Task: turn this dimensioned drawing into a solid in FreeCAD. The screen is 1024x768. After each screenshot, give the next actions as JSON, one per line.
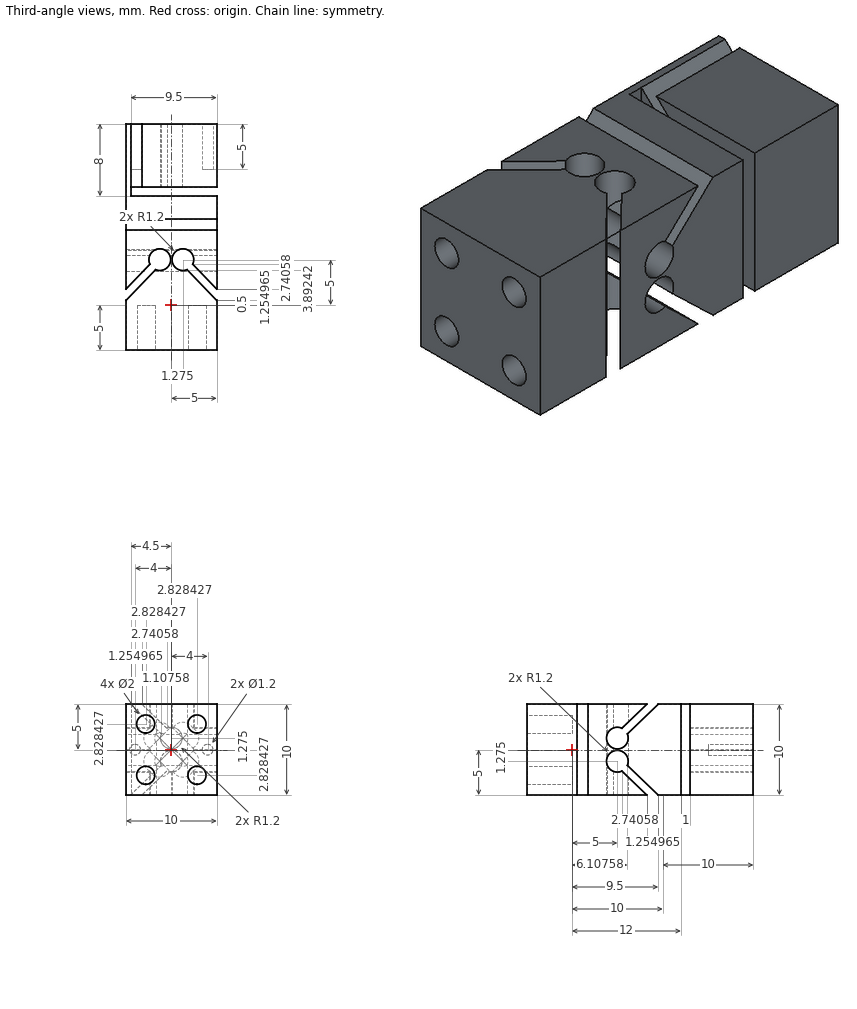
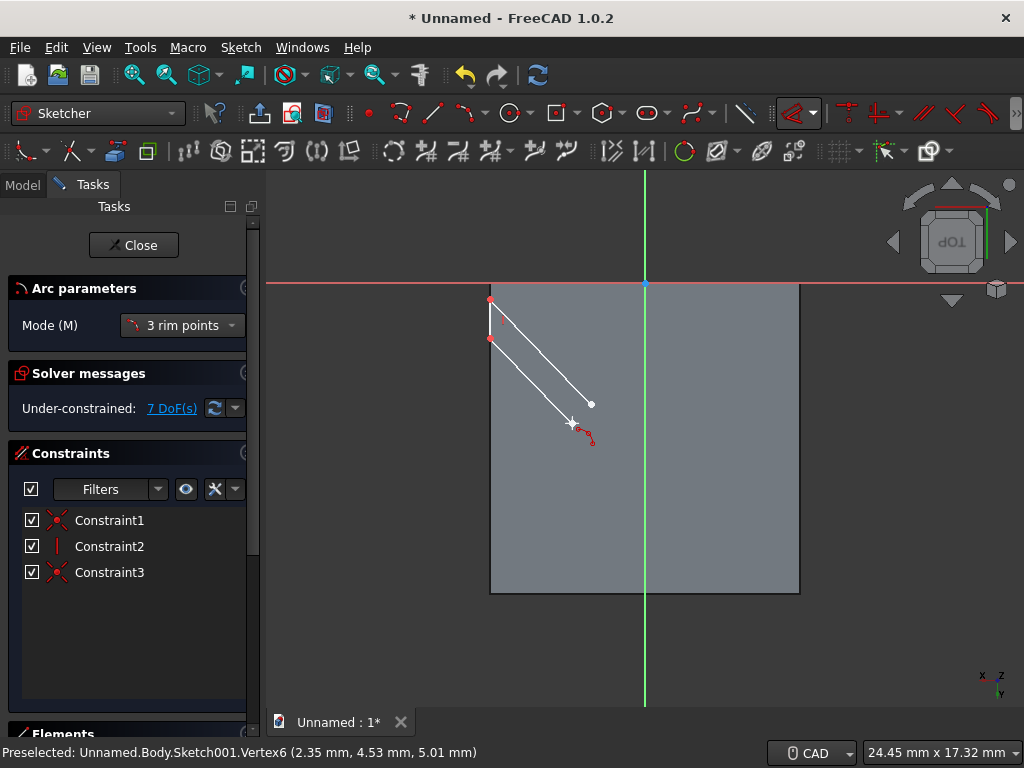
{"action": "left_click", "coordinate": [572, 424]}
{"action": "left_click", "coordinate": [591, 405]}
{"action": "left_click", "coordinate": [613, 475]}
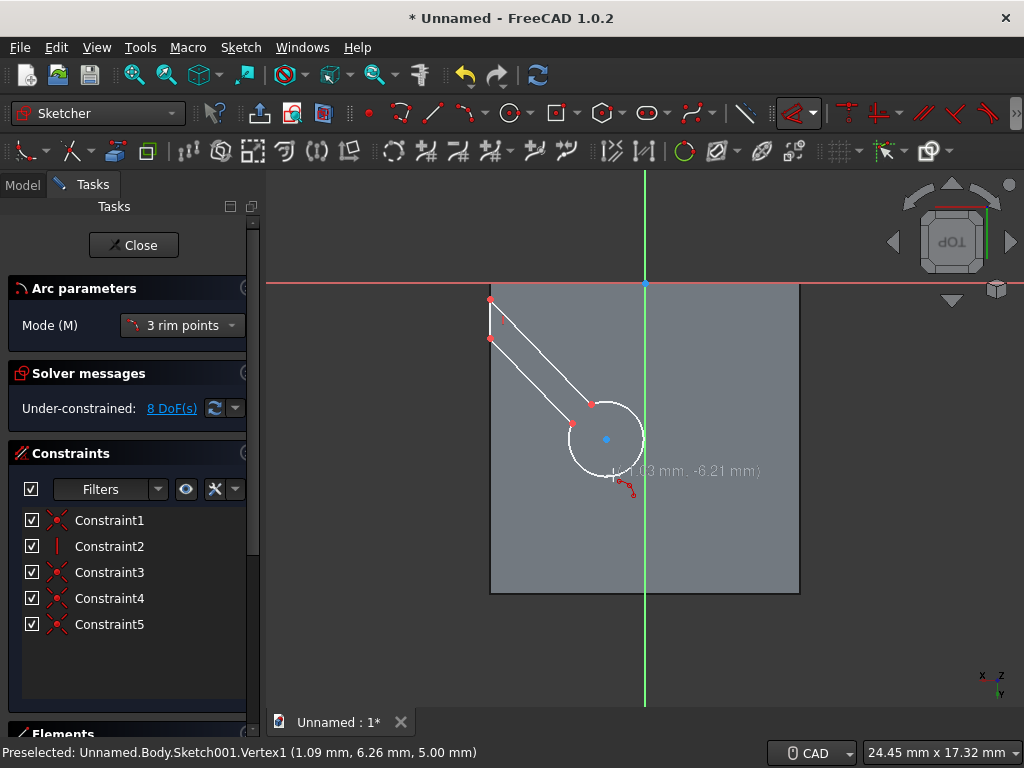
{"action": "left_click", "coordinate": [402, 114]}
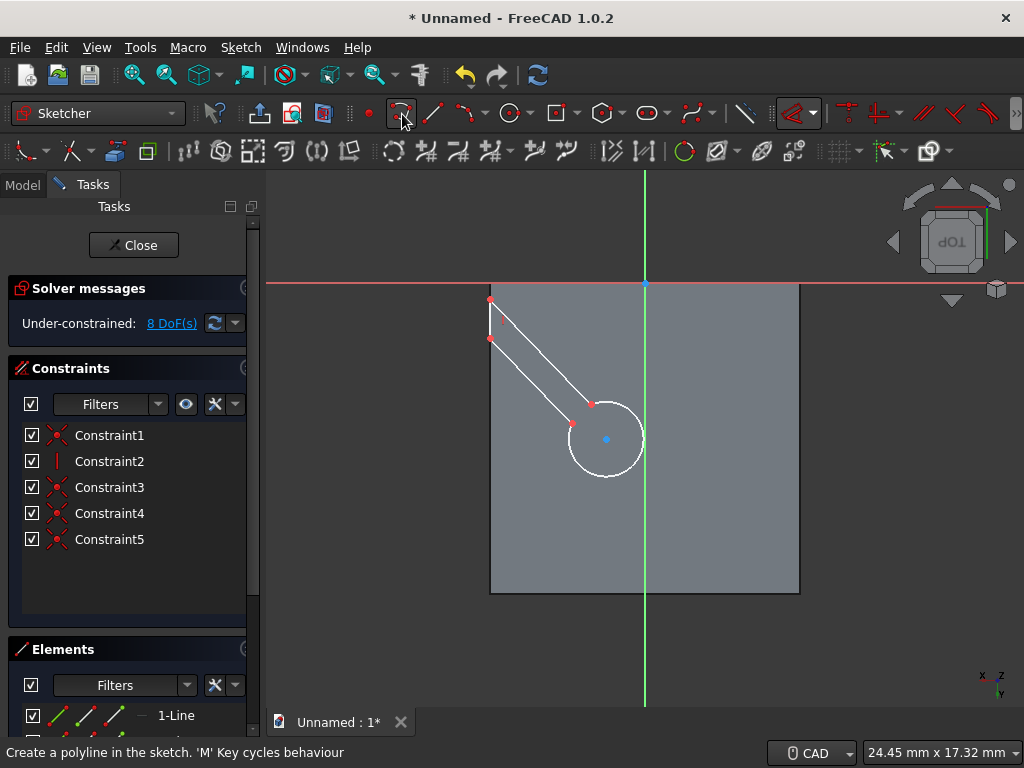
{"action": "left_click", "coordinate": [718, 423]}
{"action": "left_click", "coordinate": [800, 338]}
{"action": "left_click", "coordinate": [800, 299]}
{"action": "left_click", "coordinate": [699, 404]}
{"action": "right_click", "coordinate": [699, 404]}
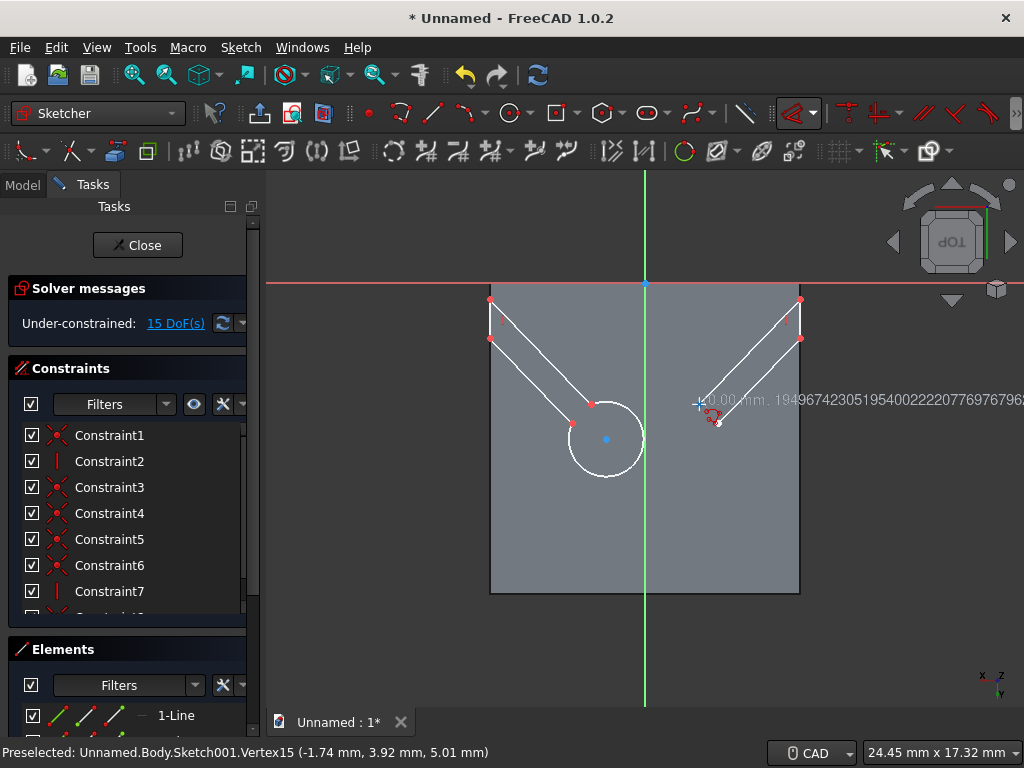
{"action": "key", "text": "g 3 a"}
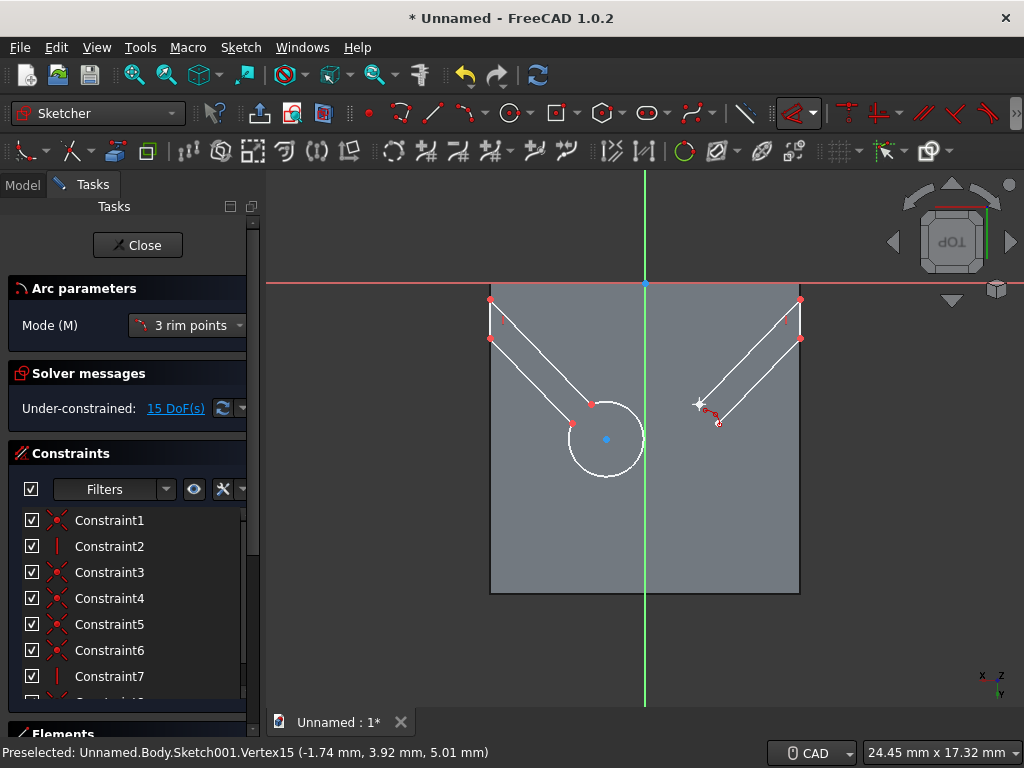
{"action": "left_click", "coordinate": [699, 405]}
{"action": "left_click", "coordinate": [718, 424]}
{"action": "left_click", "coordinate": [677, 475]}
{"action": "key", "text": "Escape"}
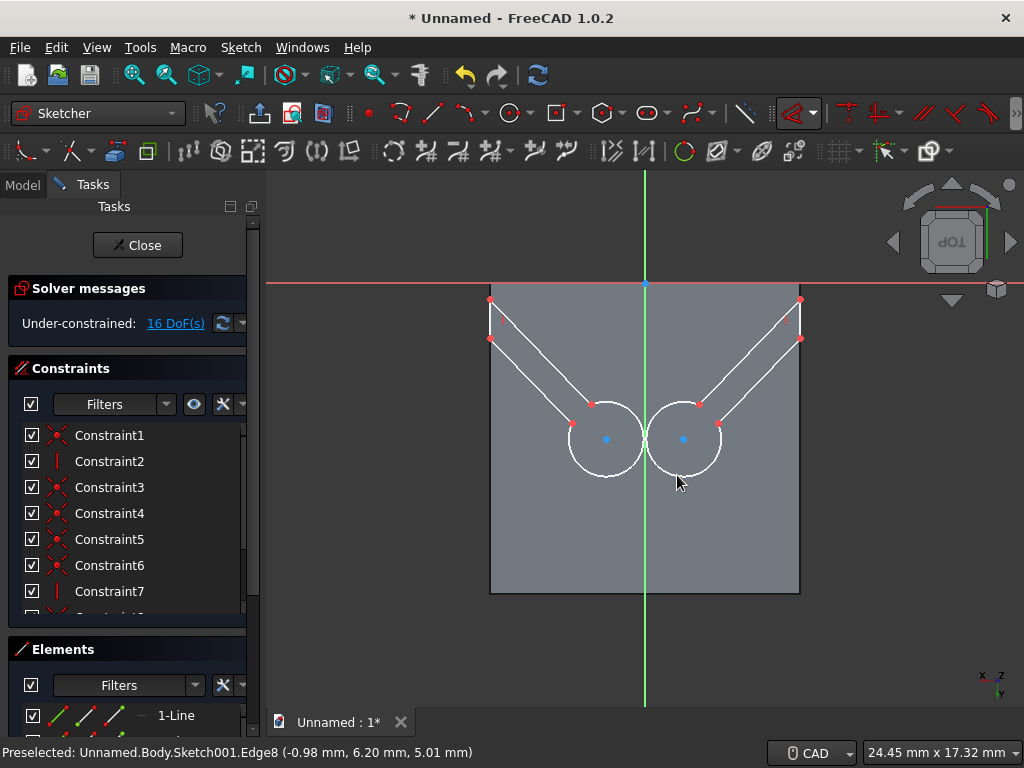
{"action": "left_click", "coordinate": [594, 475]}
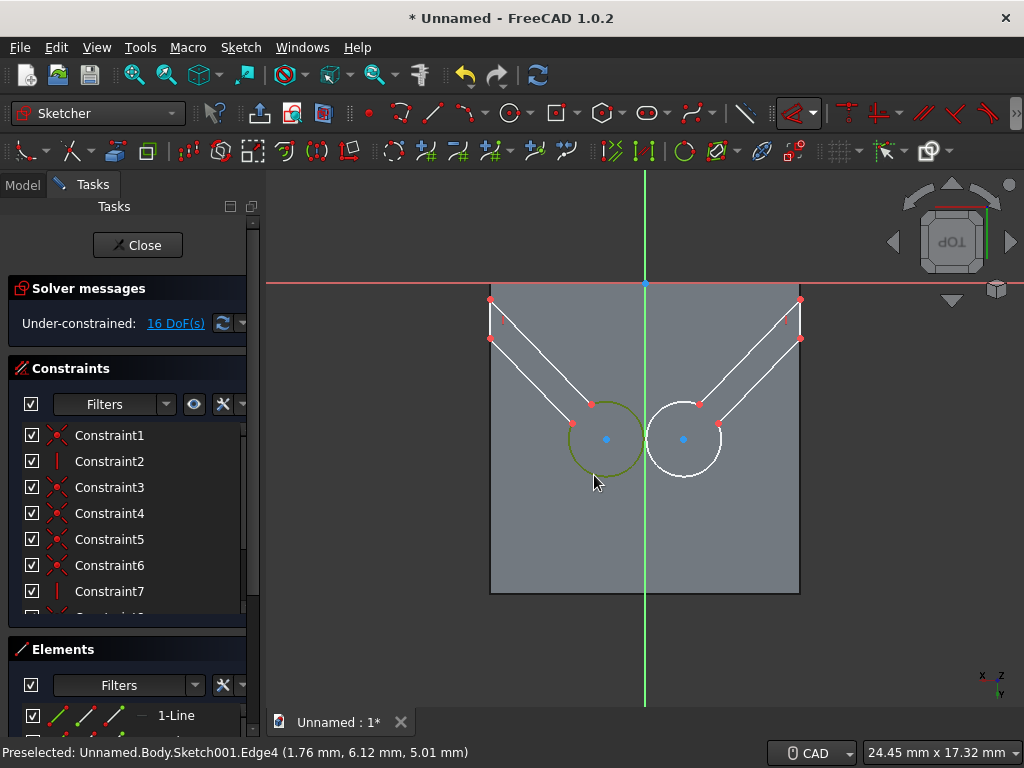
{"action": "left_click", "coordinate": [696, 475]}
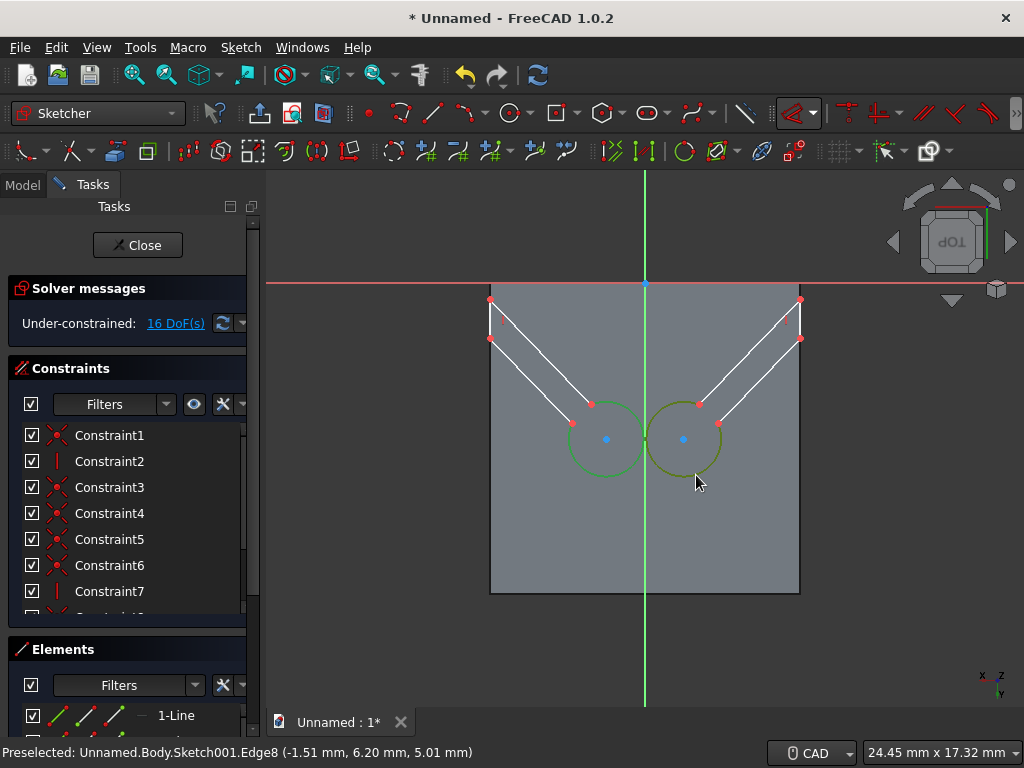
{"action": "key", "text": "e"}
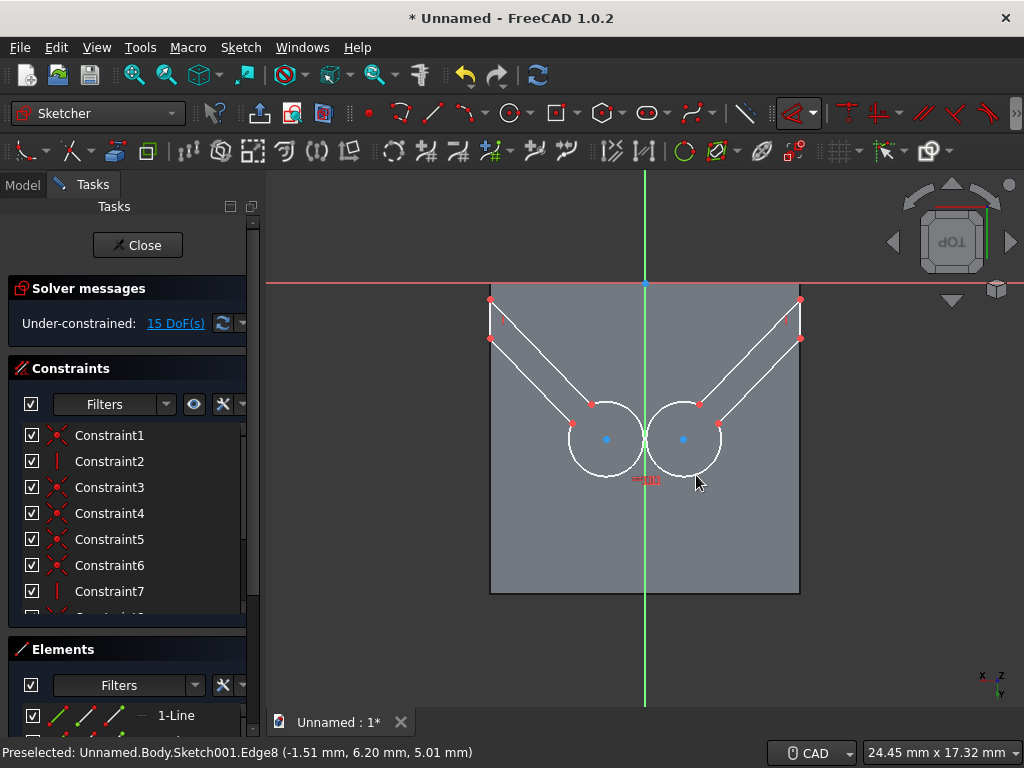
{"action": "left_click", "coordinate": [606, 439]}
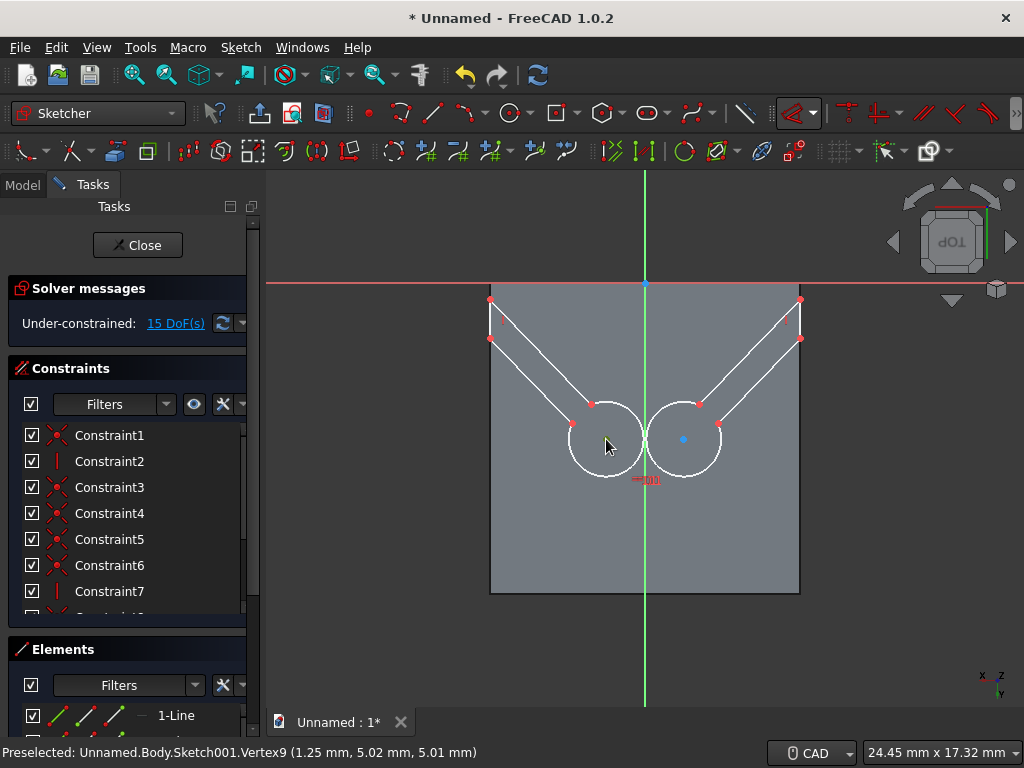
{"action": "left_click", "coordinate": [684, 439]}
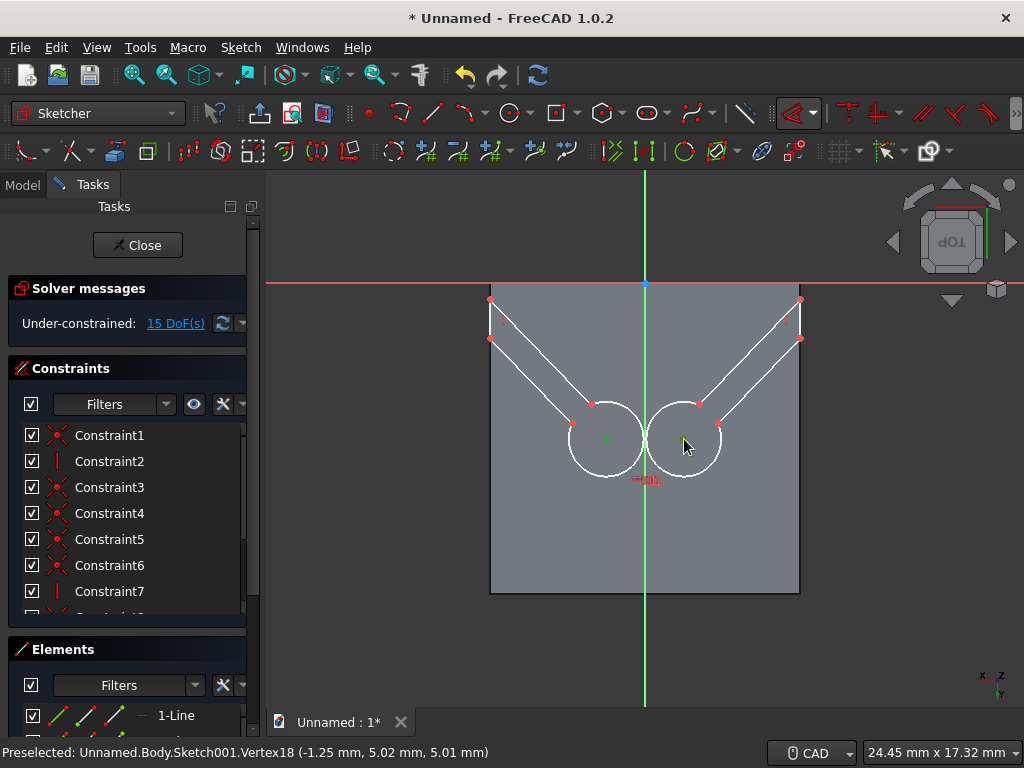
{"action": "left_click", "coordinate": [645, 645]}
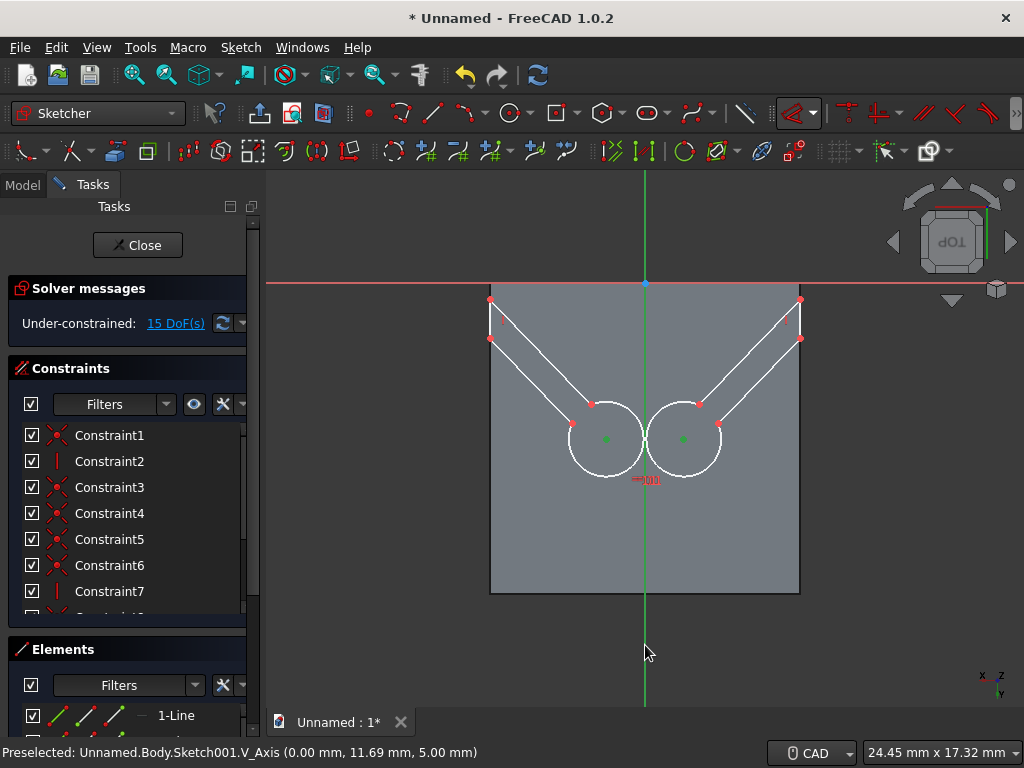
{"action": "key", "text": "s"}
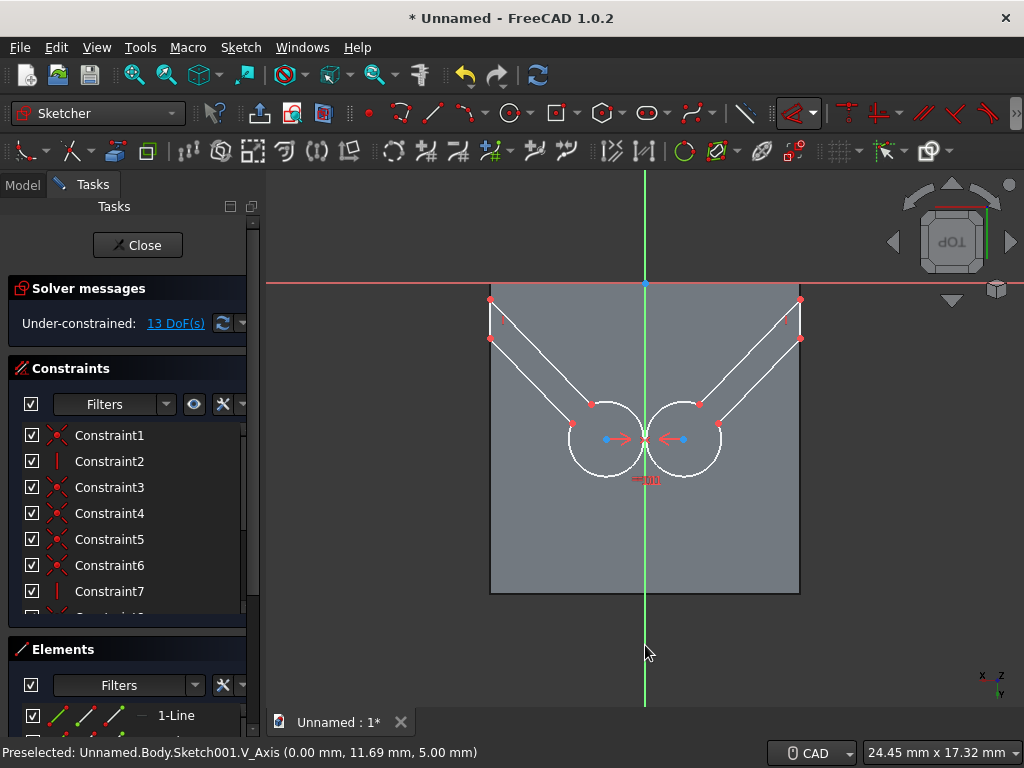
{"action": "left_click", "coordinate": [490, 339]}